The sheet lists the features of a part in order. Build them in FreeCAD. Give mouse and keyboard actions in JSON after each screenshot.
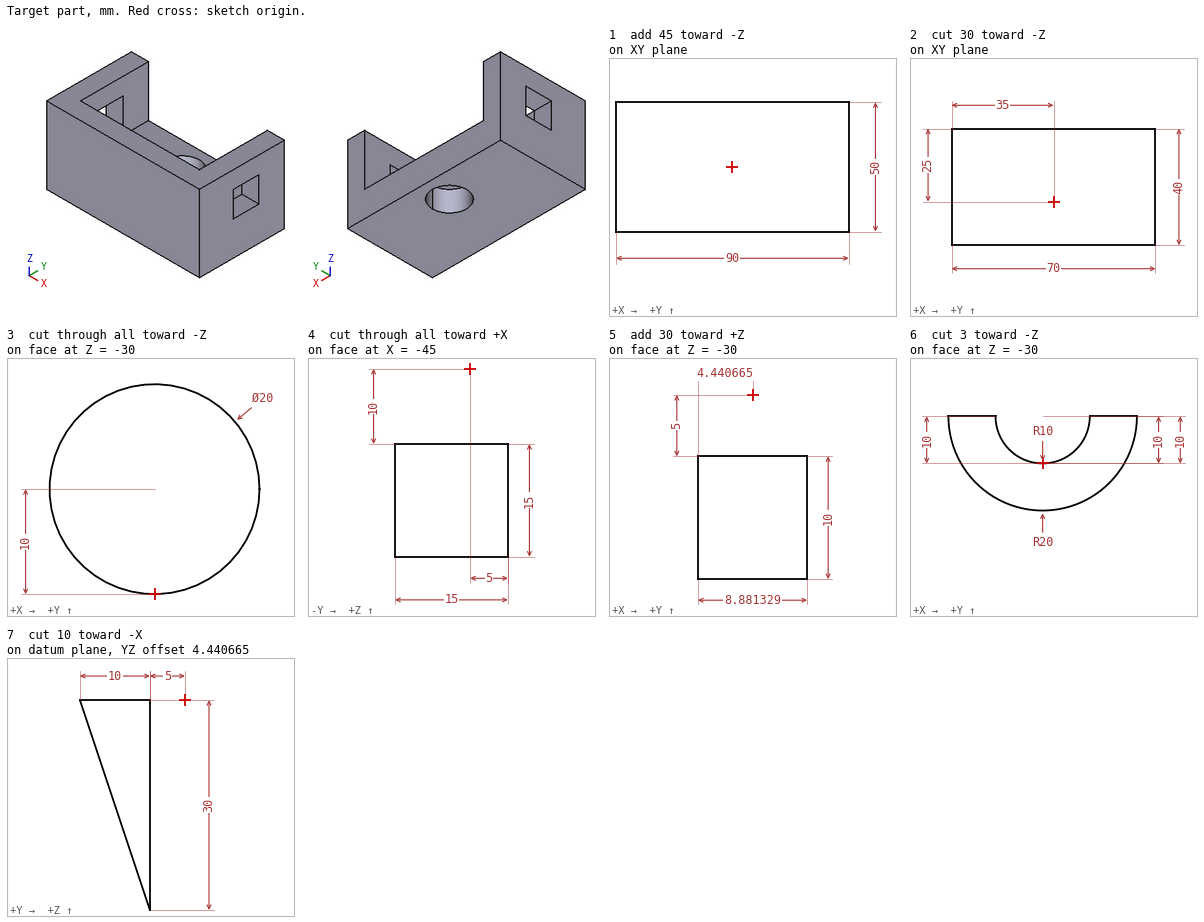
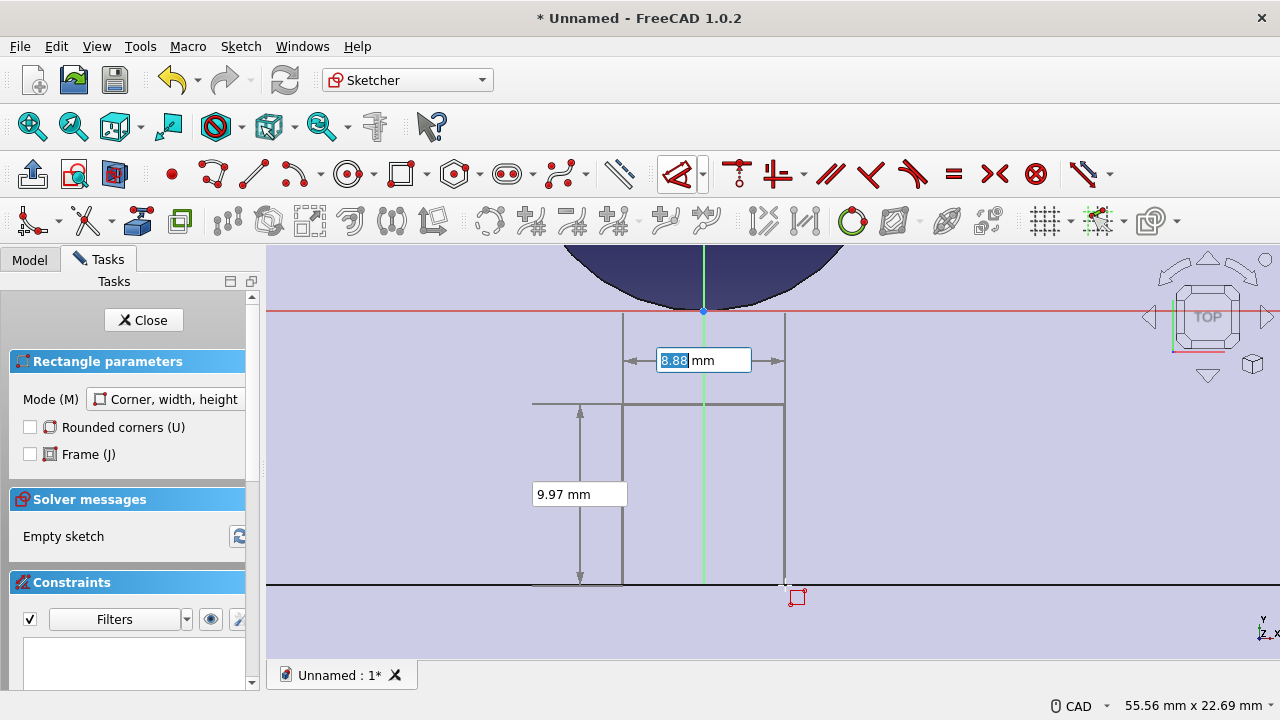
{"action": "type", "text": "8.881329"}
{"action": "key", "text": "Tab"}
{"action": "type", "text": "10"}
{"action": "key", "text": "Return"}
{"action": "key", "text": "Escape"}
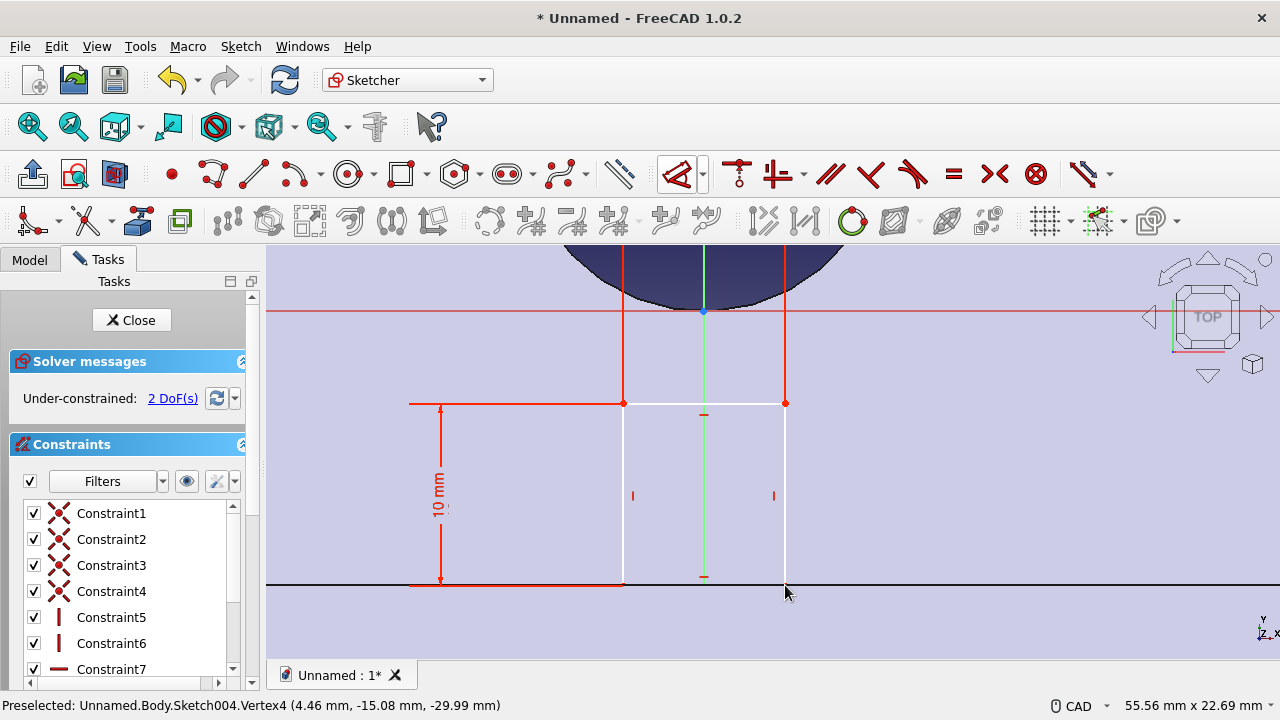
{"action": "left_click", "coordinate": [623, 404]}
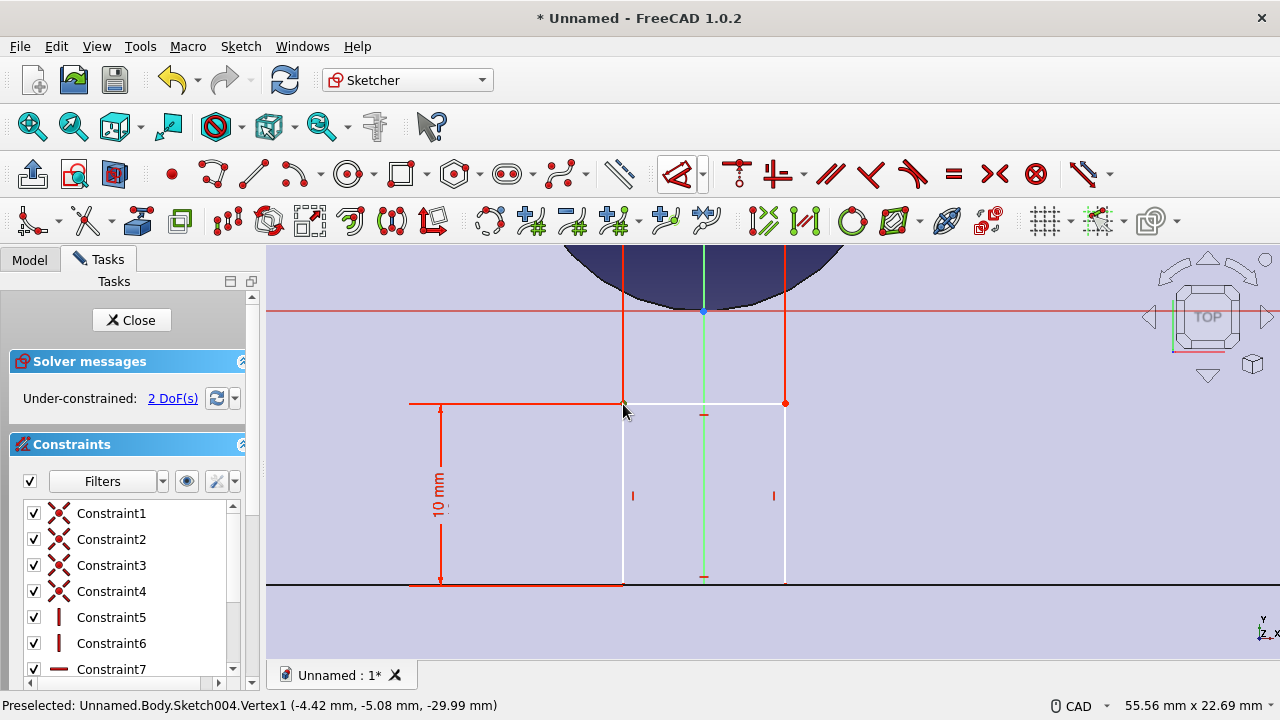
{"action": "key", "text": "i"}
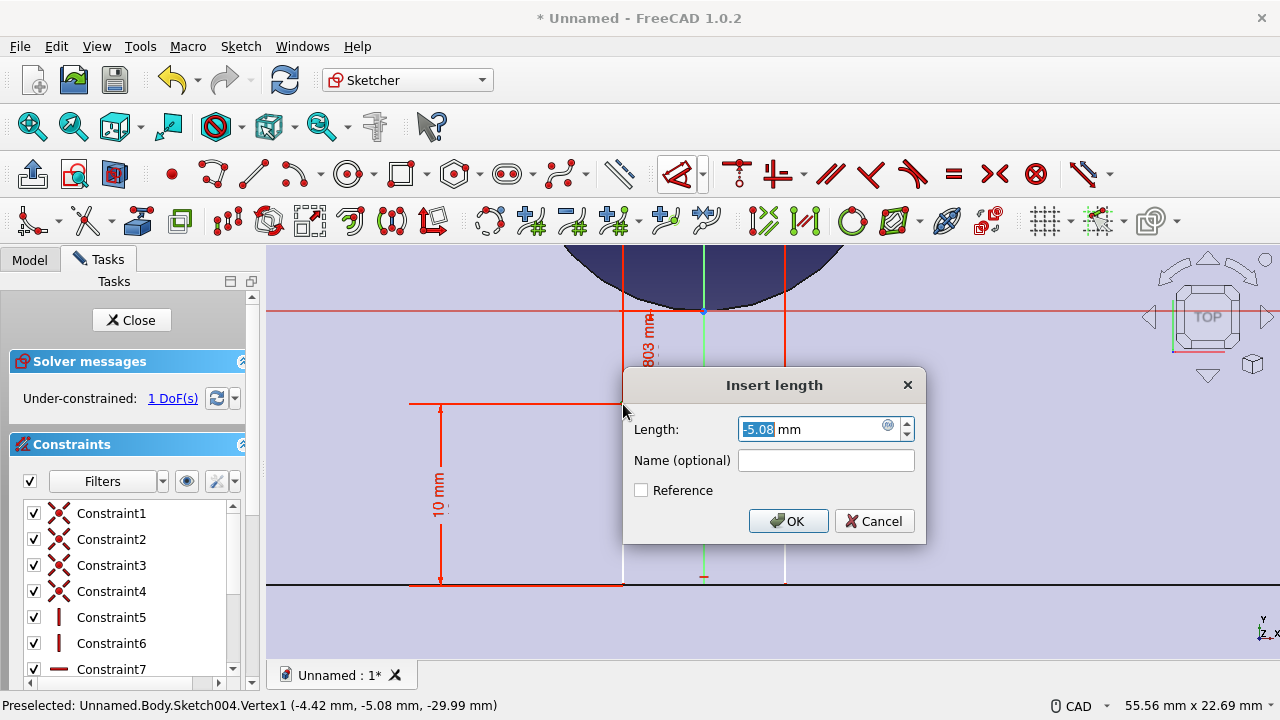
{"action": "type", "text": "-5"}
{"action": "key", "text": "Return"}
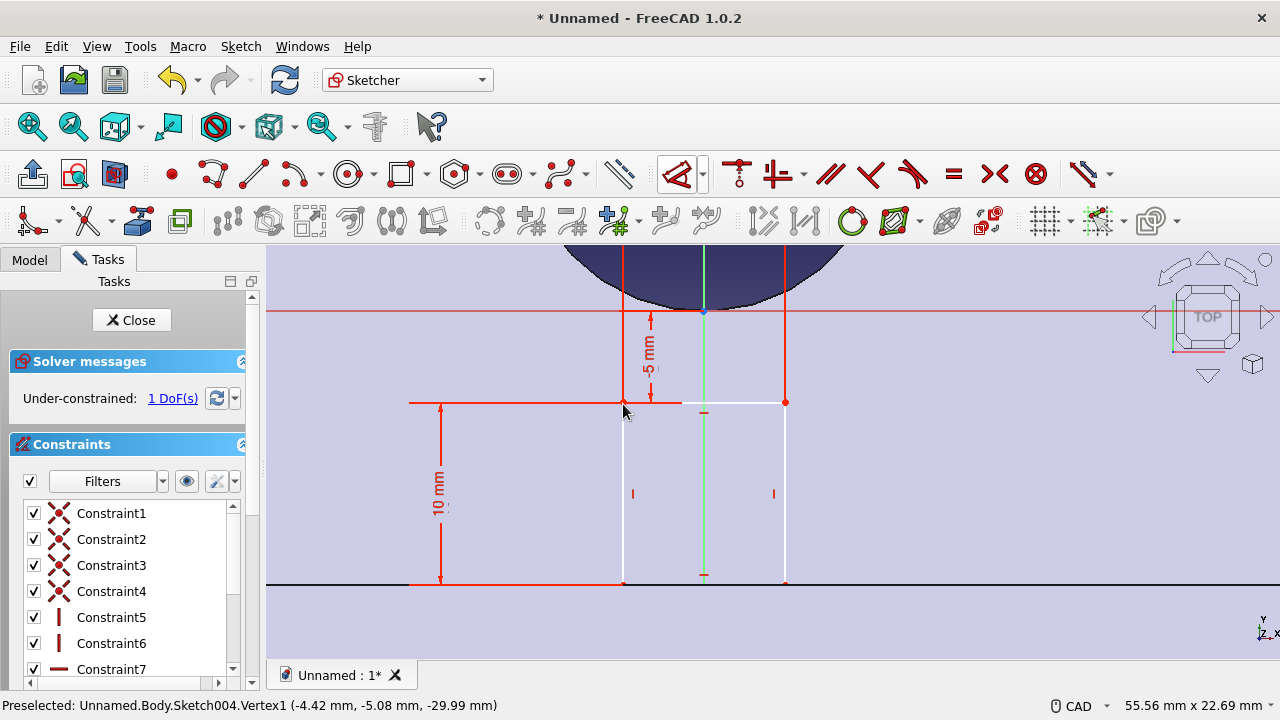
{"action": "left_click", "coordinate": [623, 403]}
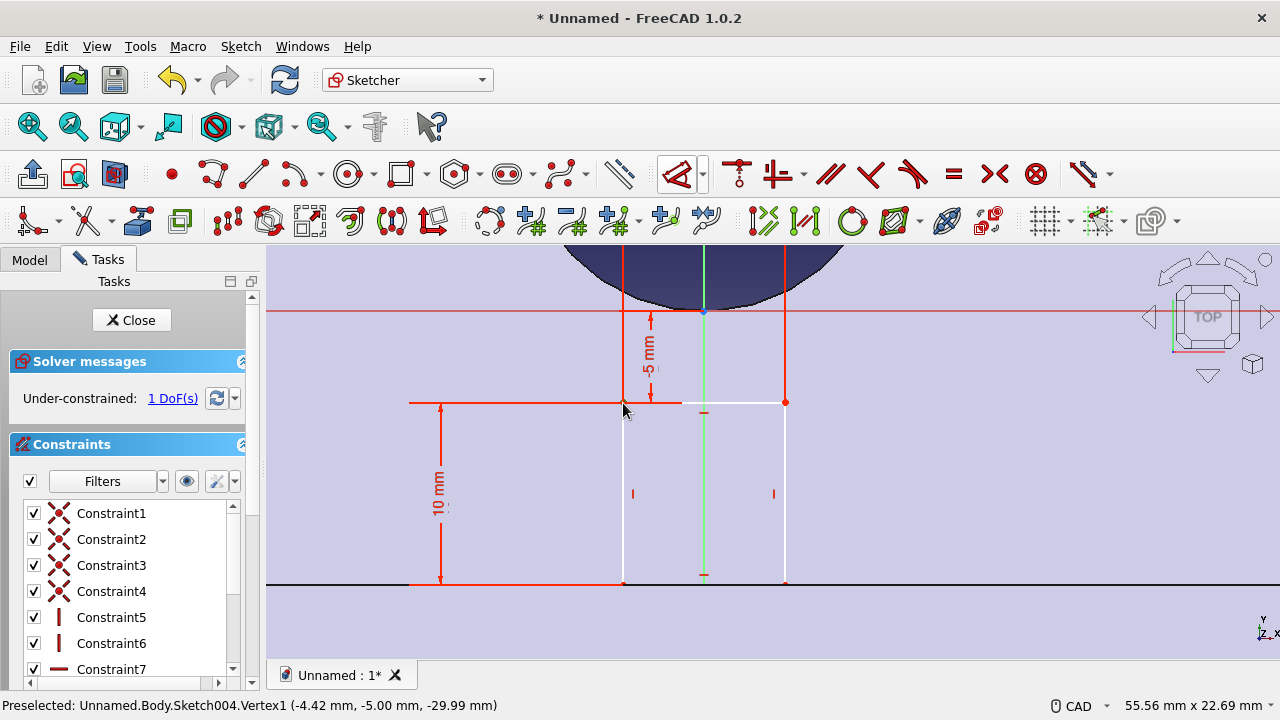
{"action": "key", "text": "l"}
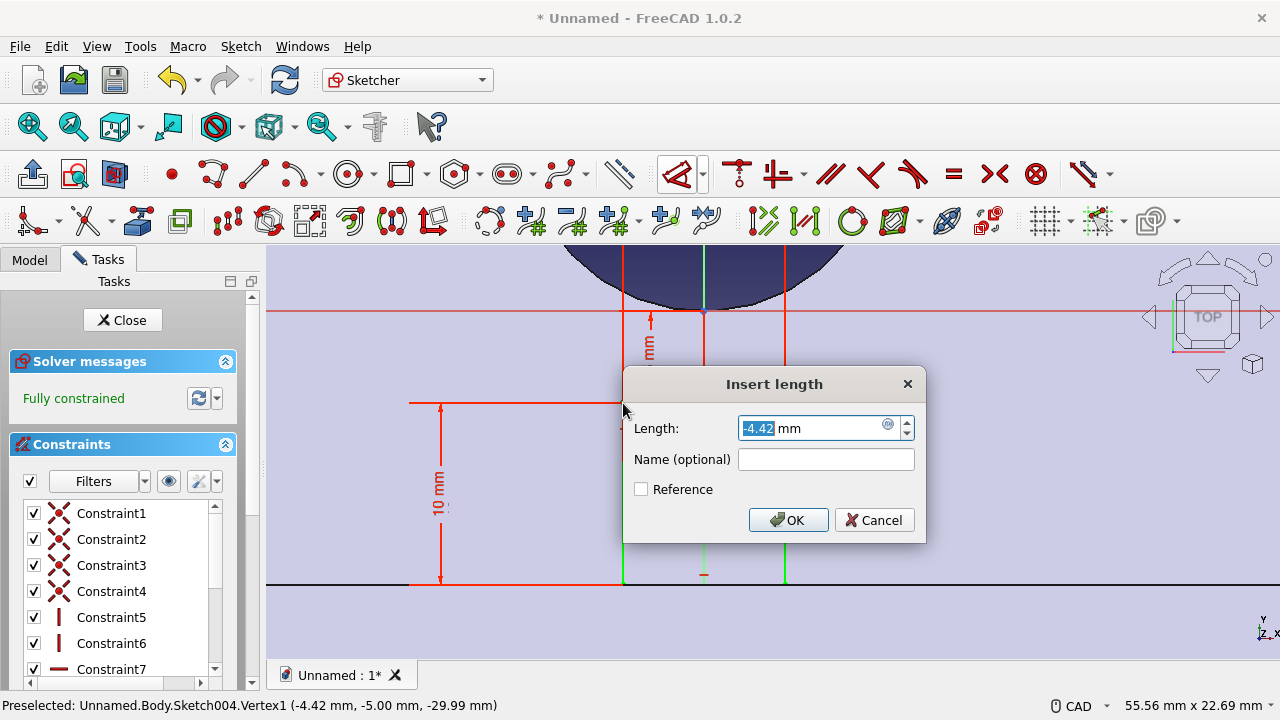
{"action": "type", "text": "-4.440665"}
{"action": "key", "text": "Return"}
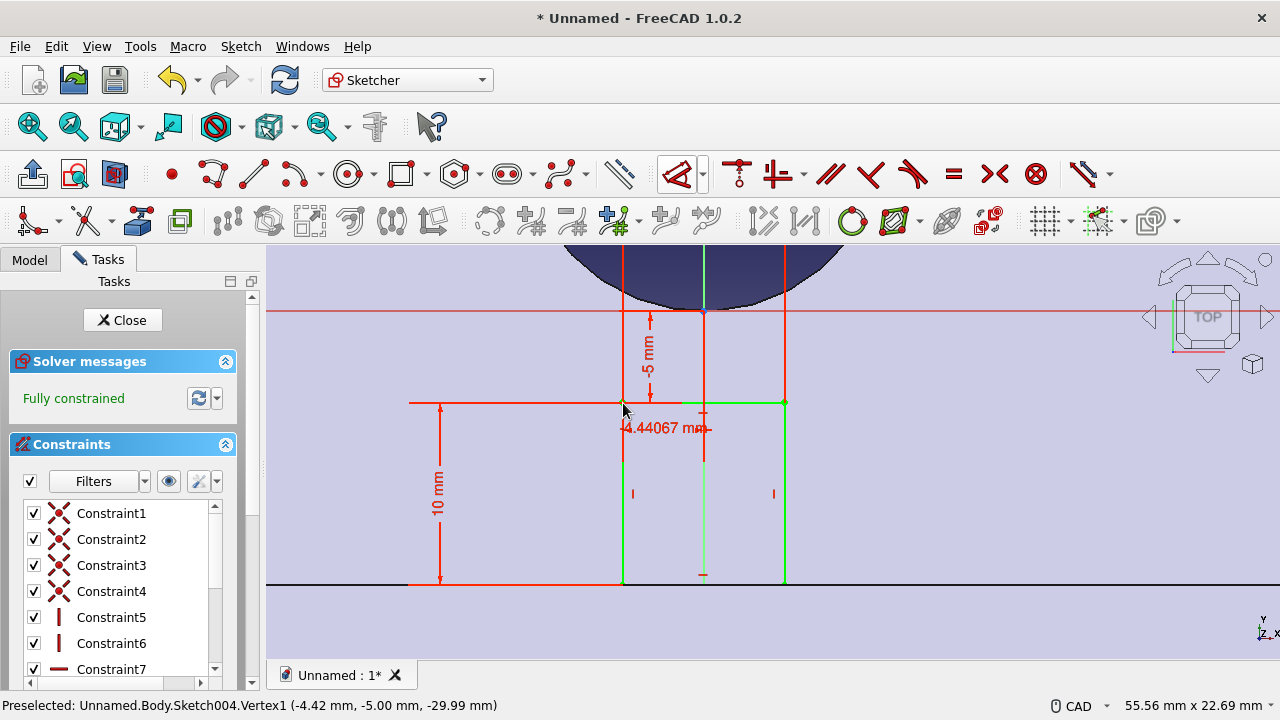
{"action": "left_click", "coordinate": [123, 320]}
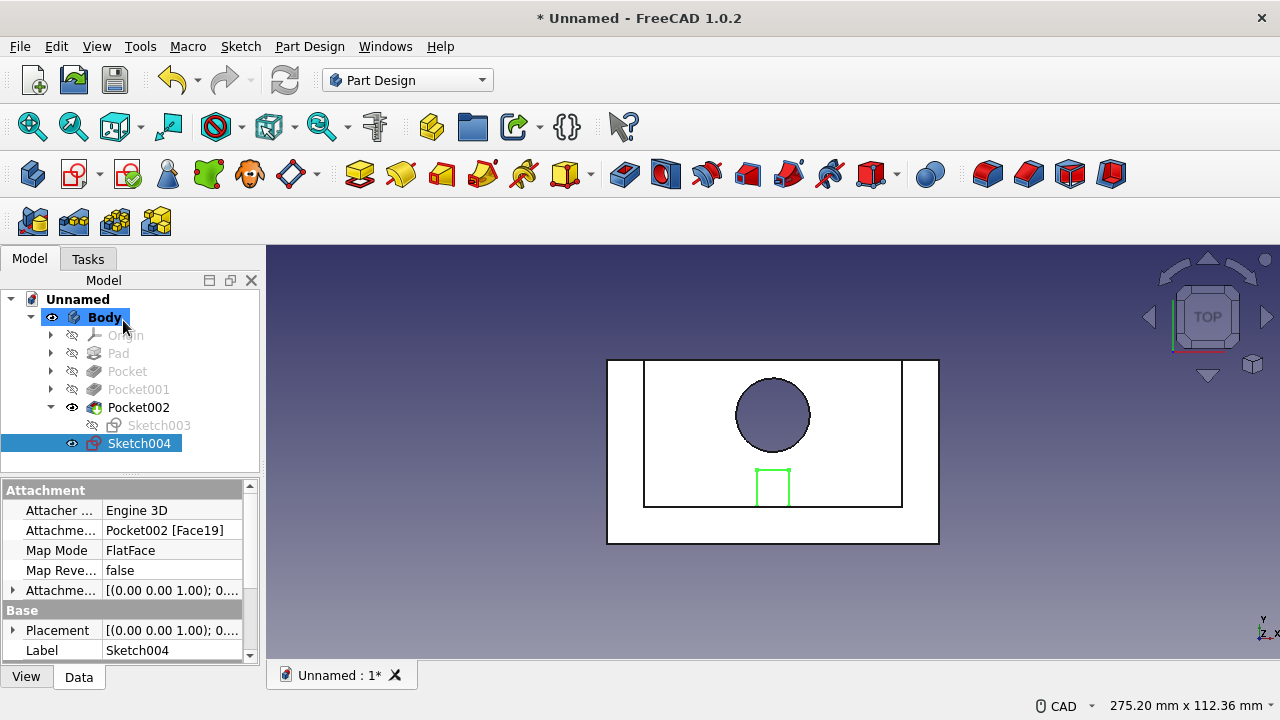
{"action": "left_click", "coordinate": [360, 174]}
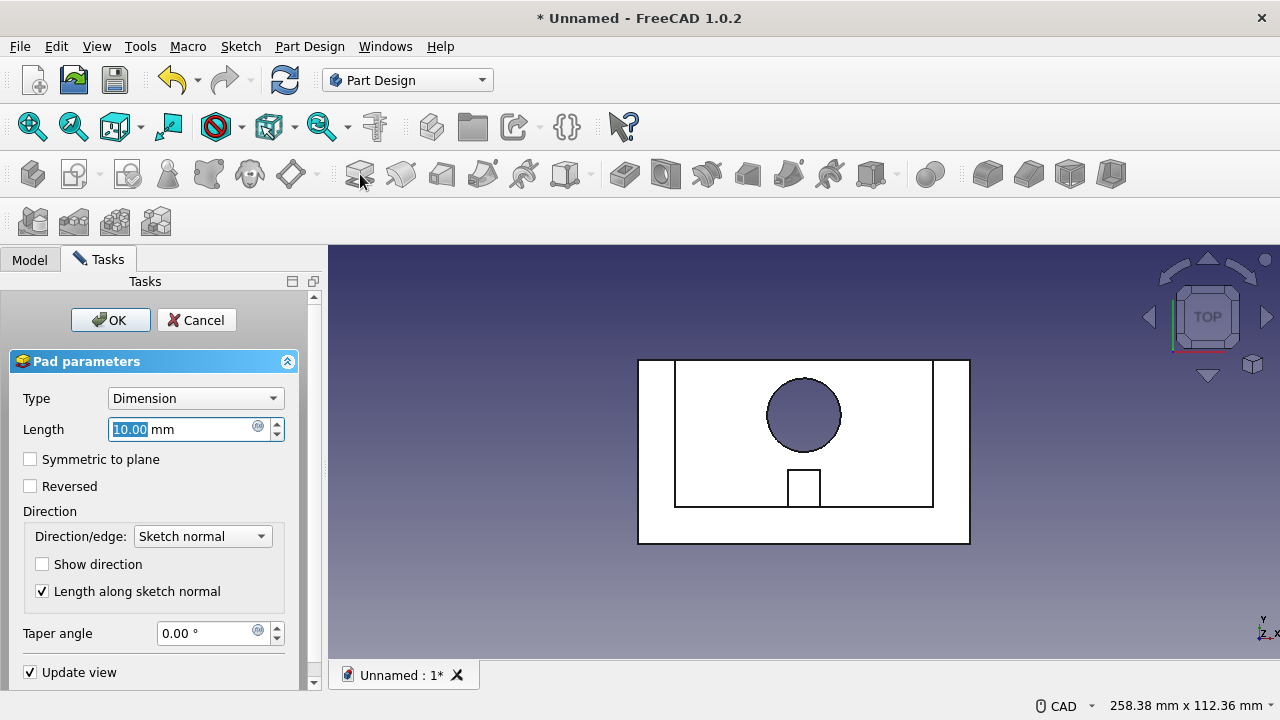
{"action": "type", "text": "30"}
{"action": "key", "text": "Tab"}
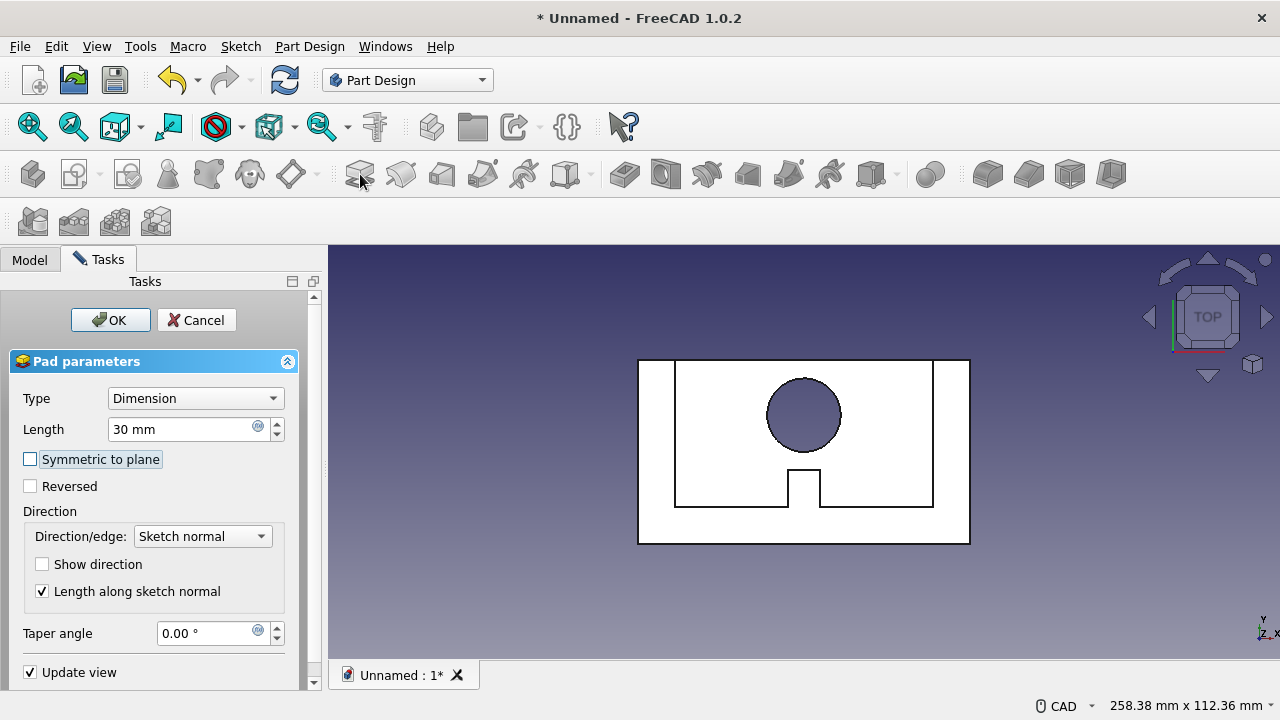
{"action": "left_click", "coordinate": [111, 320]}